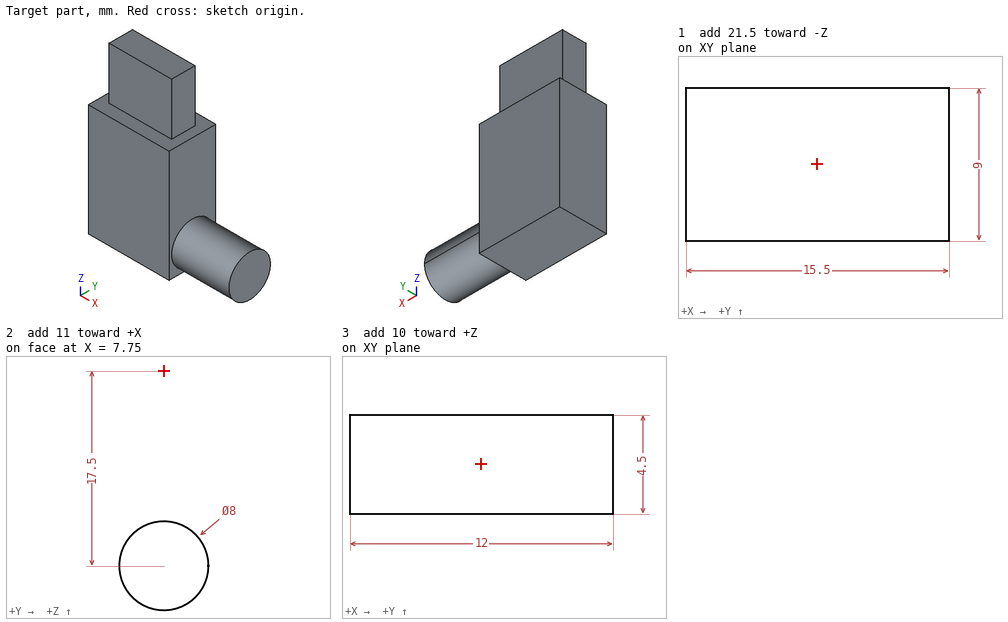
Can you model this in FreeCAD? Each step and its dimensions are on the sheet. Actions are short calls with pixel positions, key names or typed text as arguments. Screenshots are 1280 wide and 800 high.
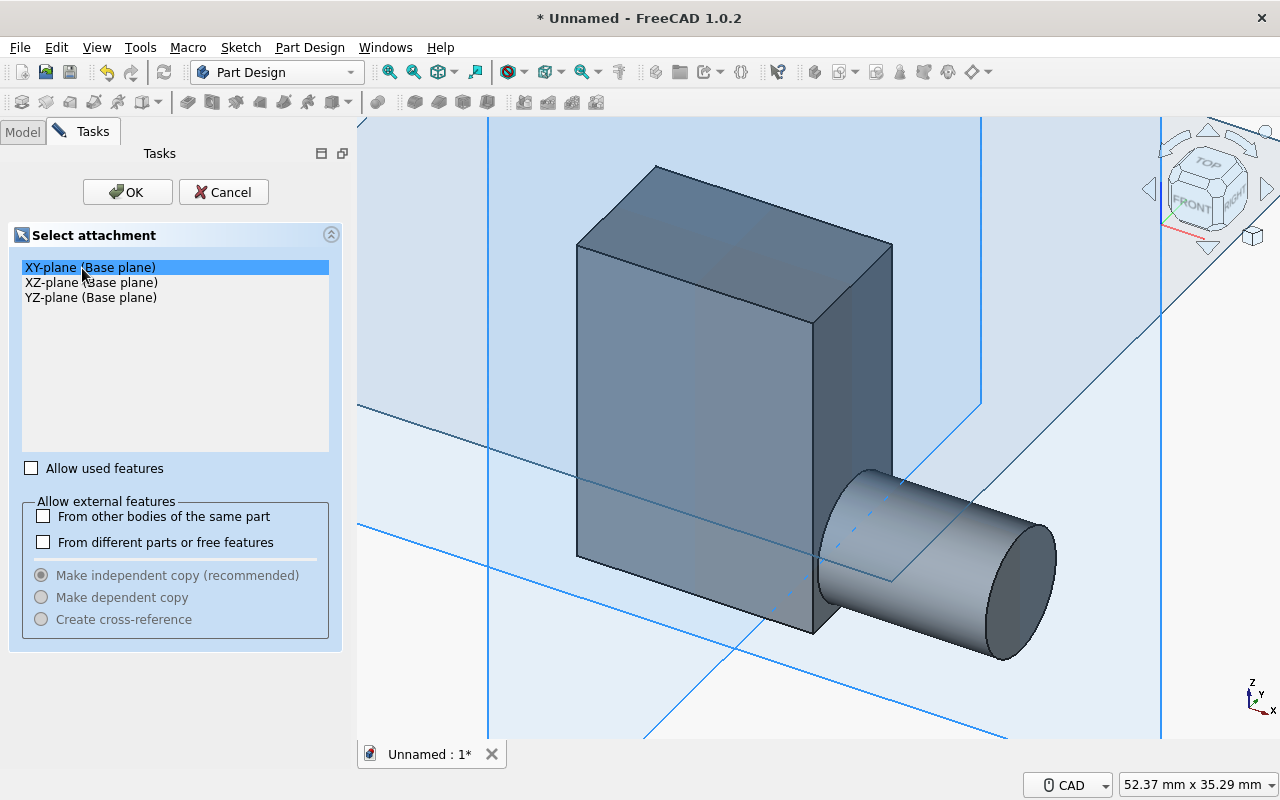
click(128, 192)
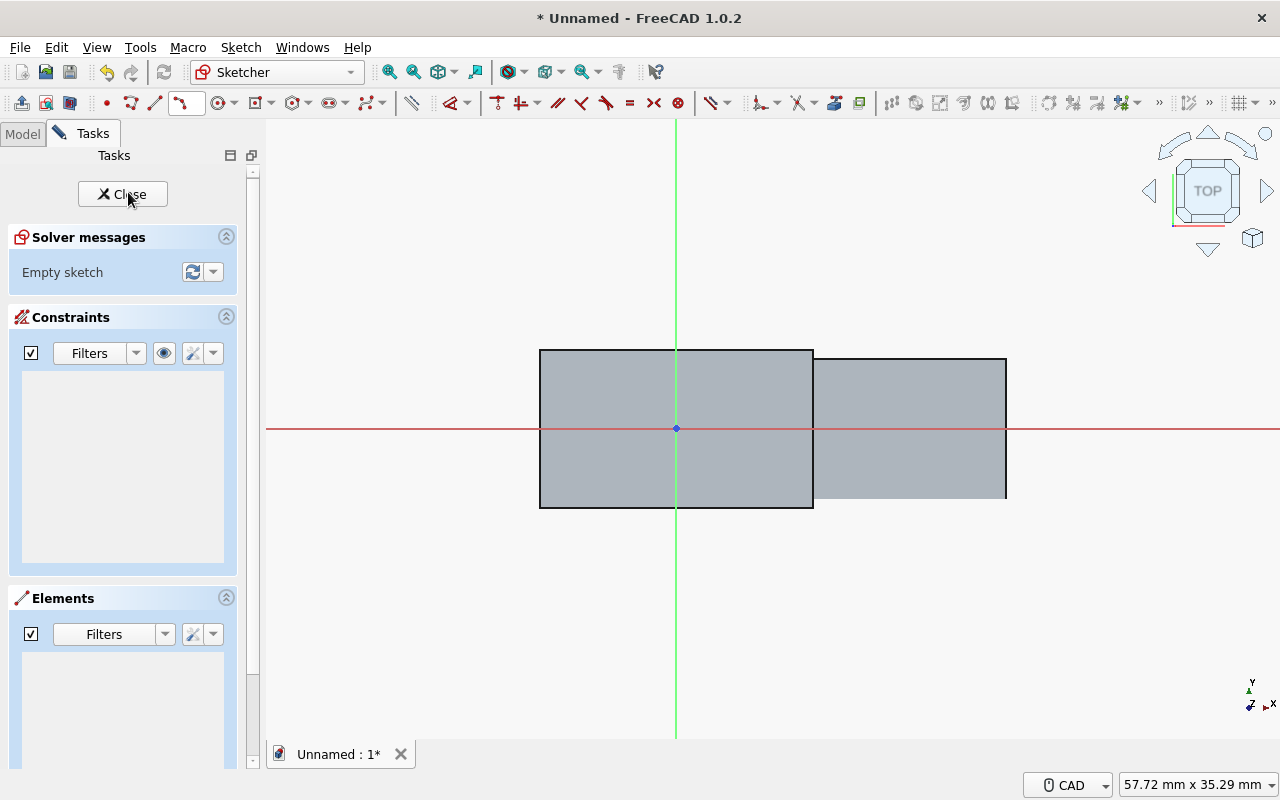
scroll(660, 429, up, 5)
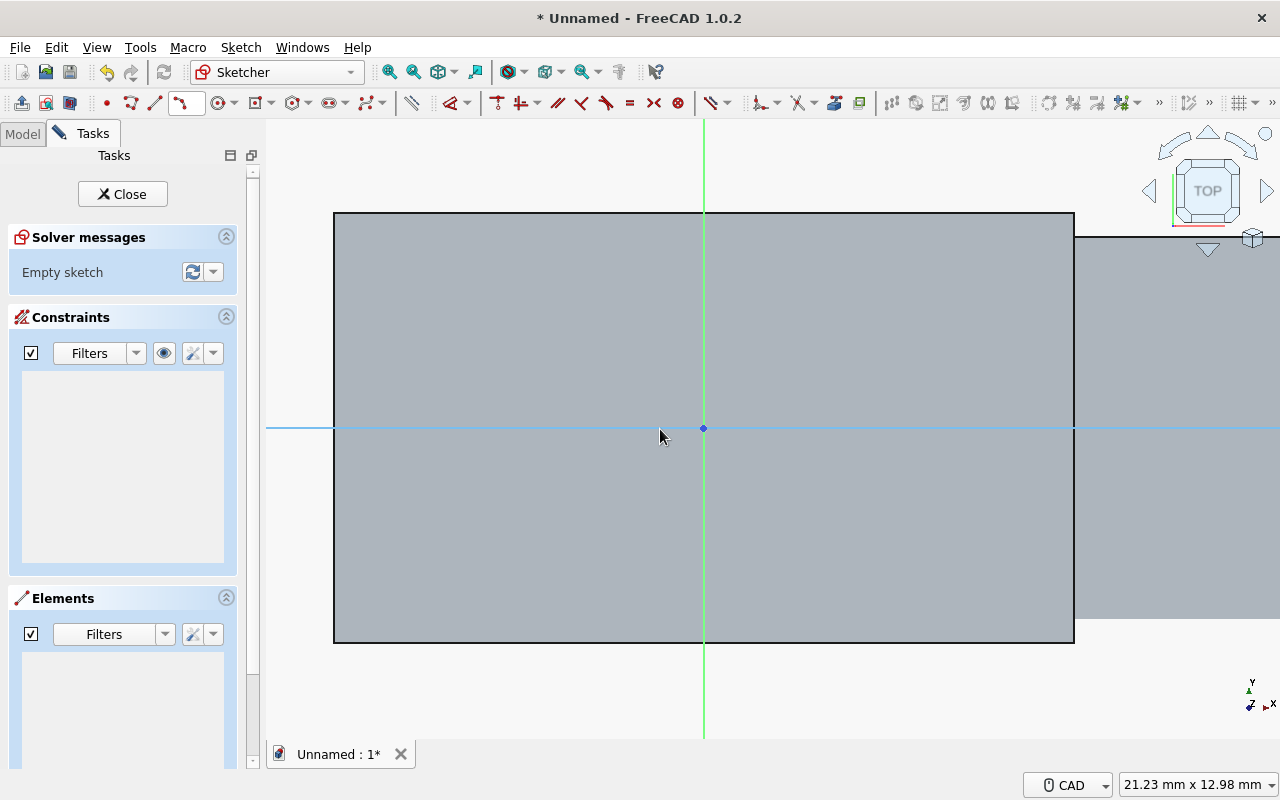
click(256, 104)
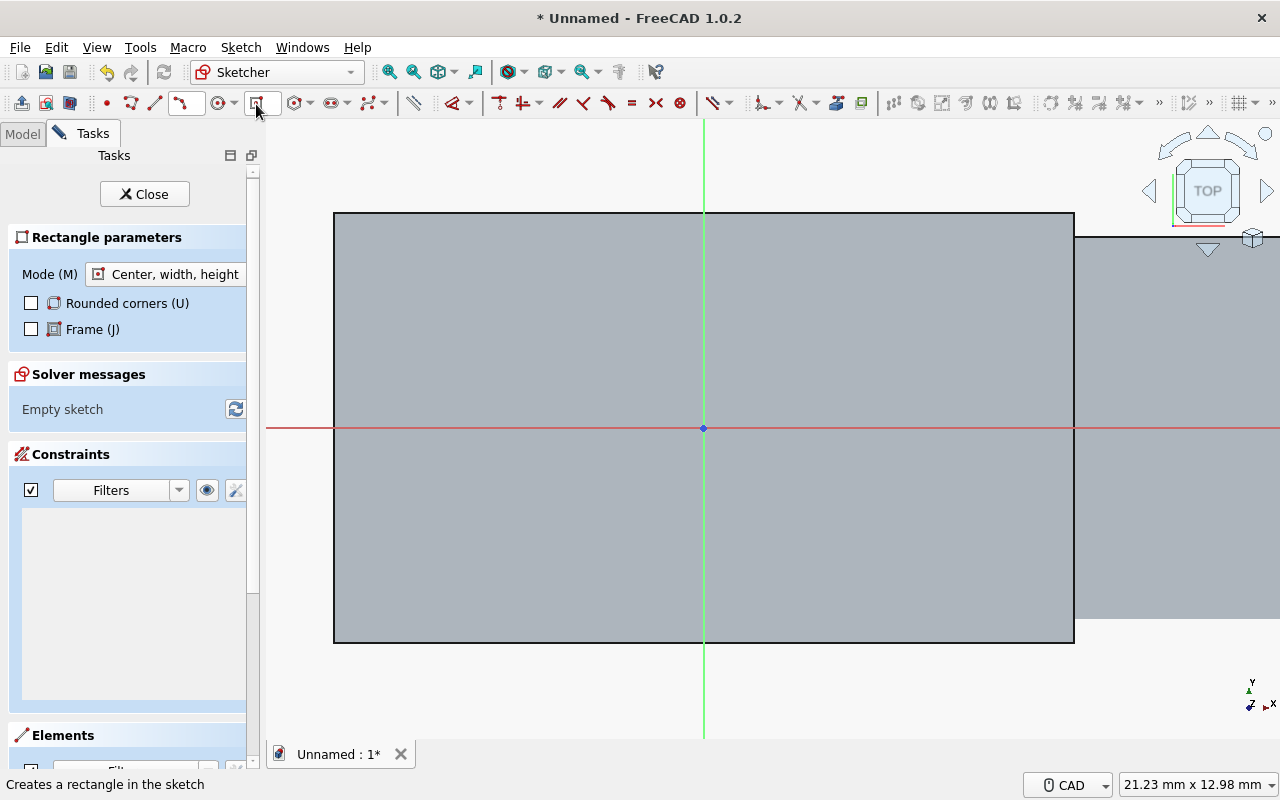
click(704, 428)
move(990, 321)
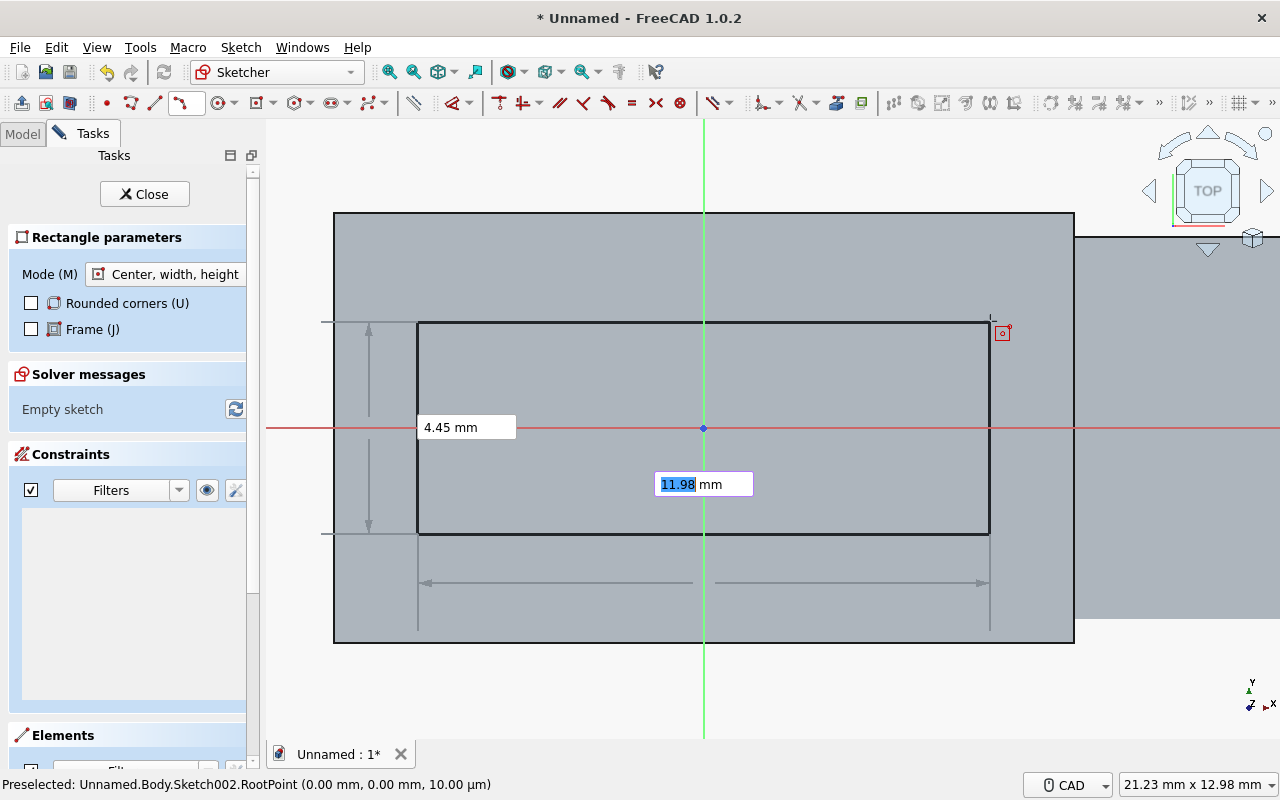
text(12)
key(Tab)
text(4.5)
key(Return)
key(Escape)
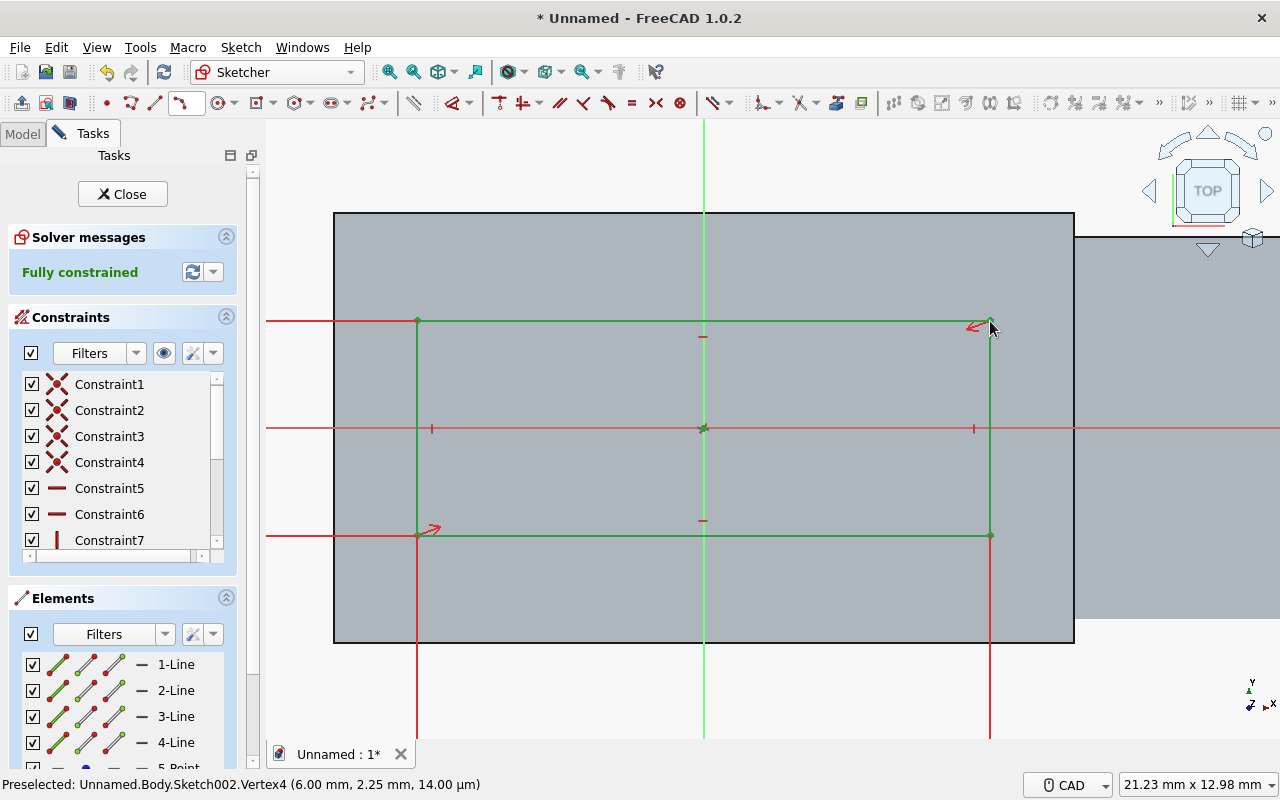
click(123, 194)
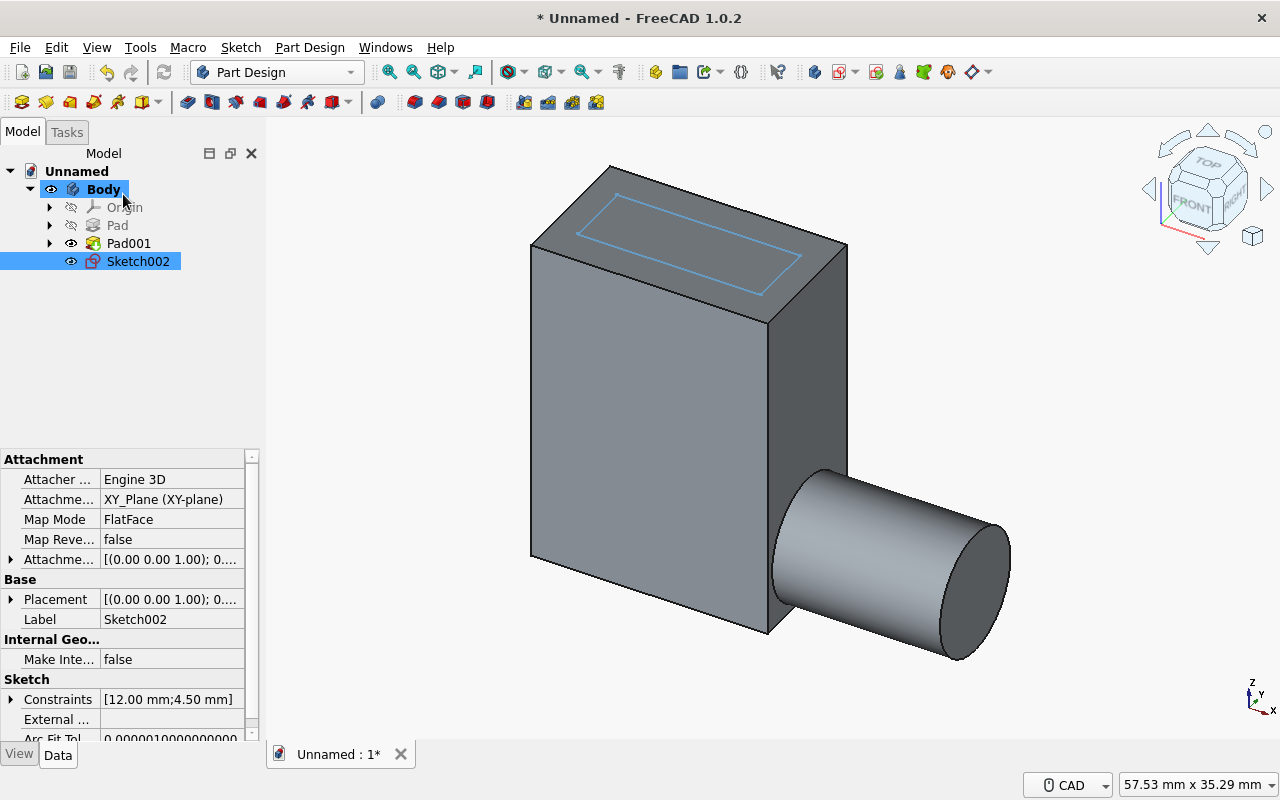
click(22, 102)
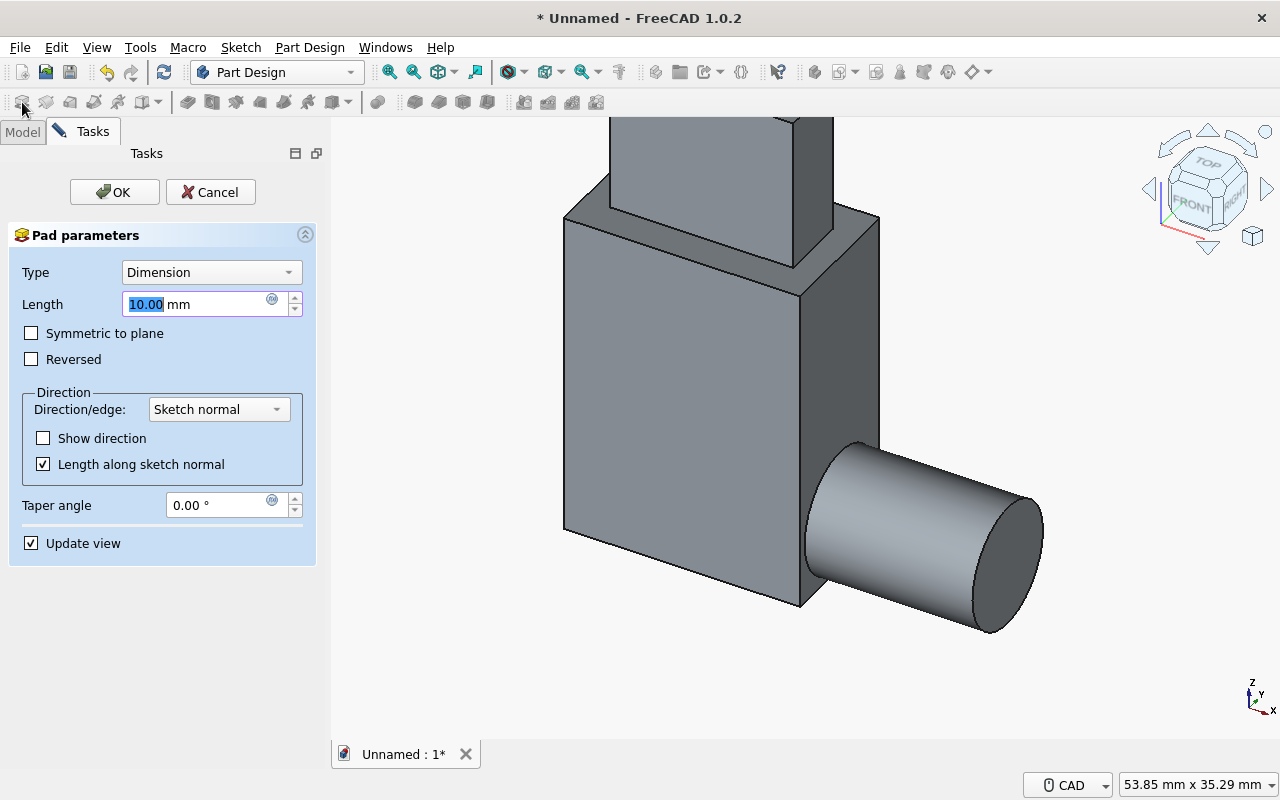
text(10)
key(Tab)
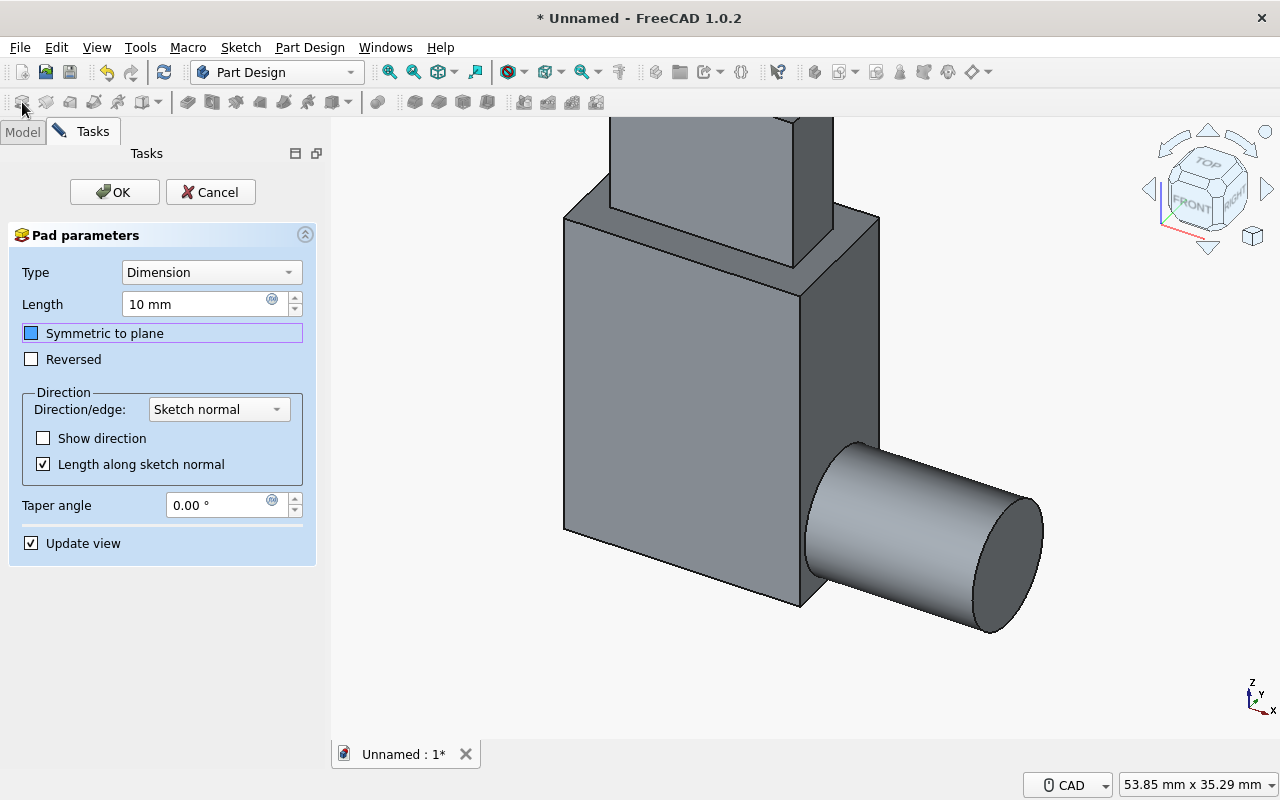
click(115, 192)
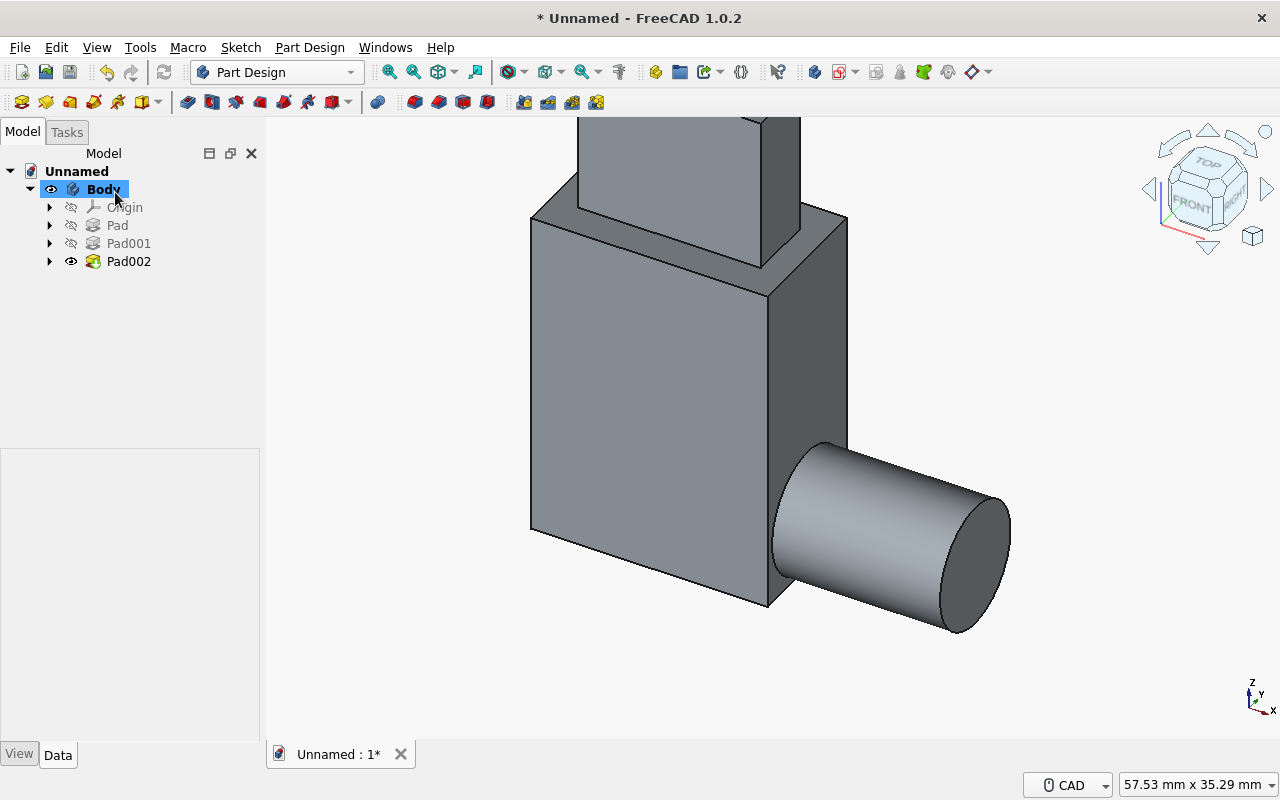
key(0)